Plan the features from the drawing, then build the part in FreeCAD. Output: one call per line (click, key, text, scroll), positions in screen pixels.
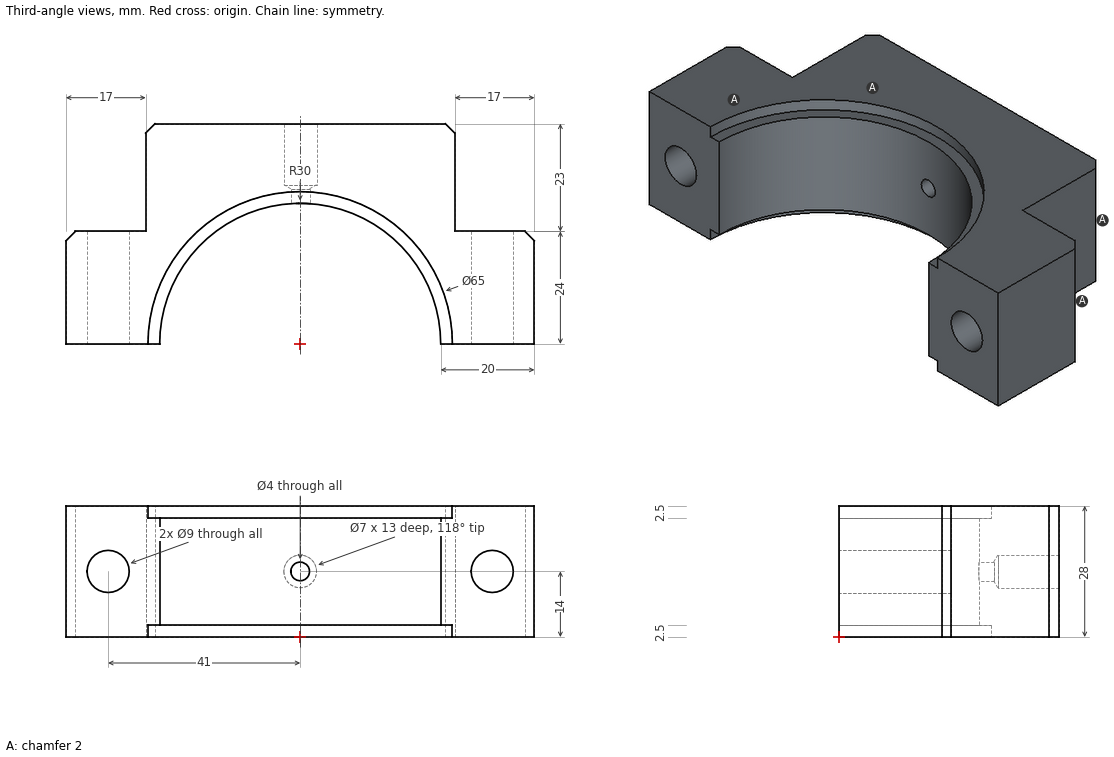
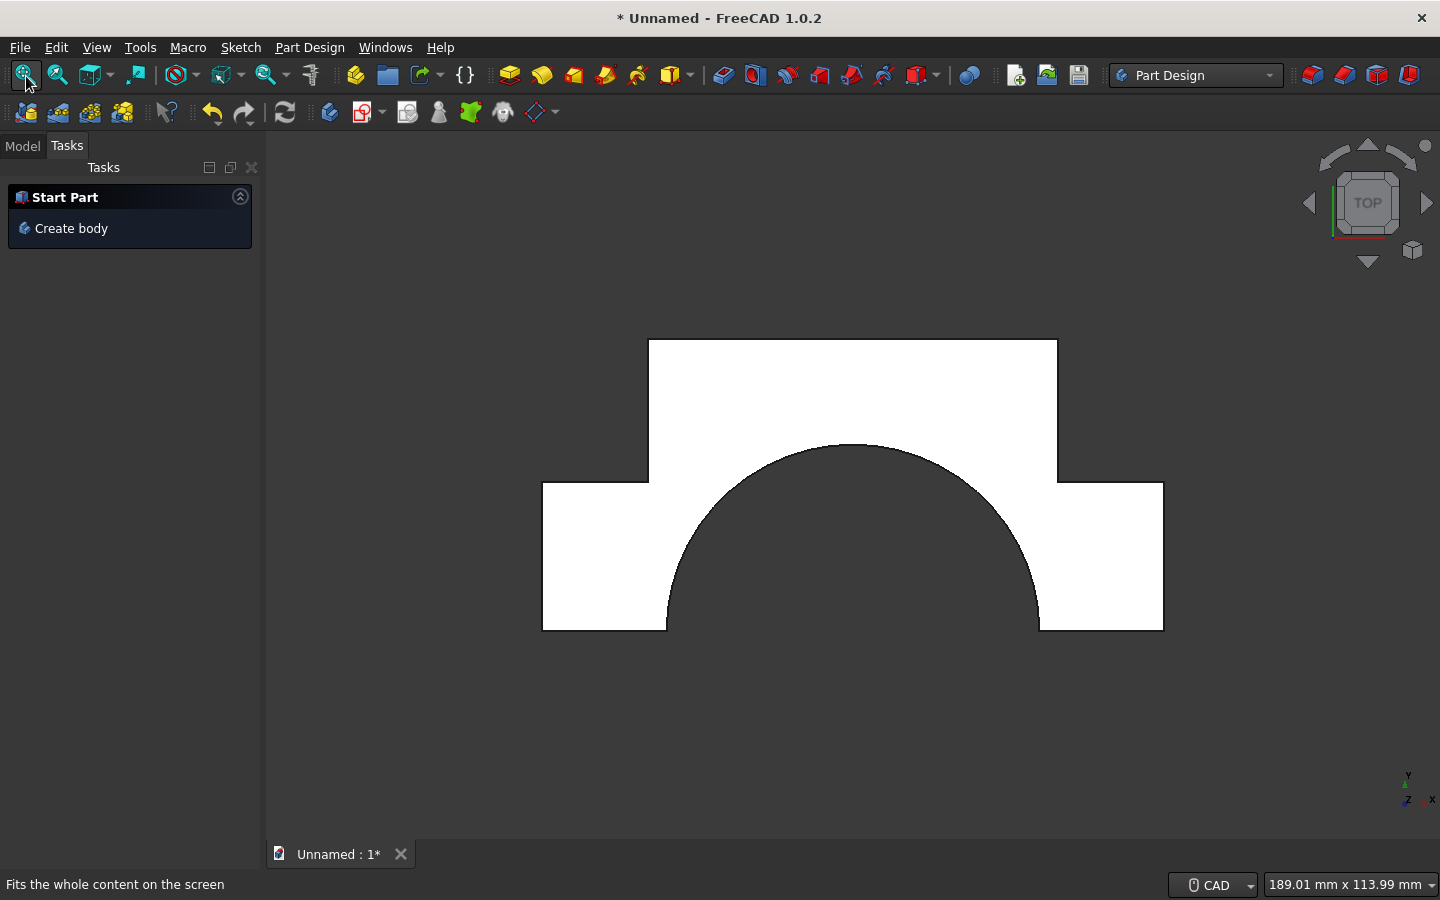
key(1)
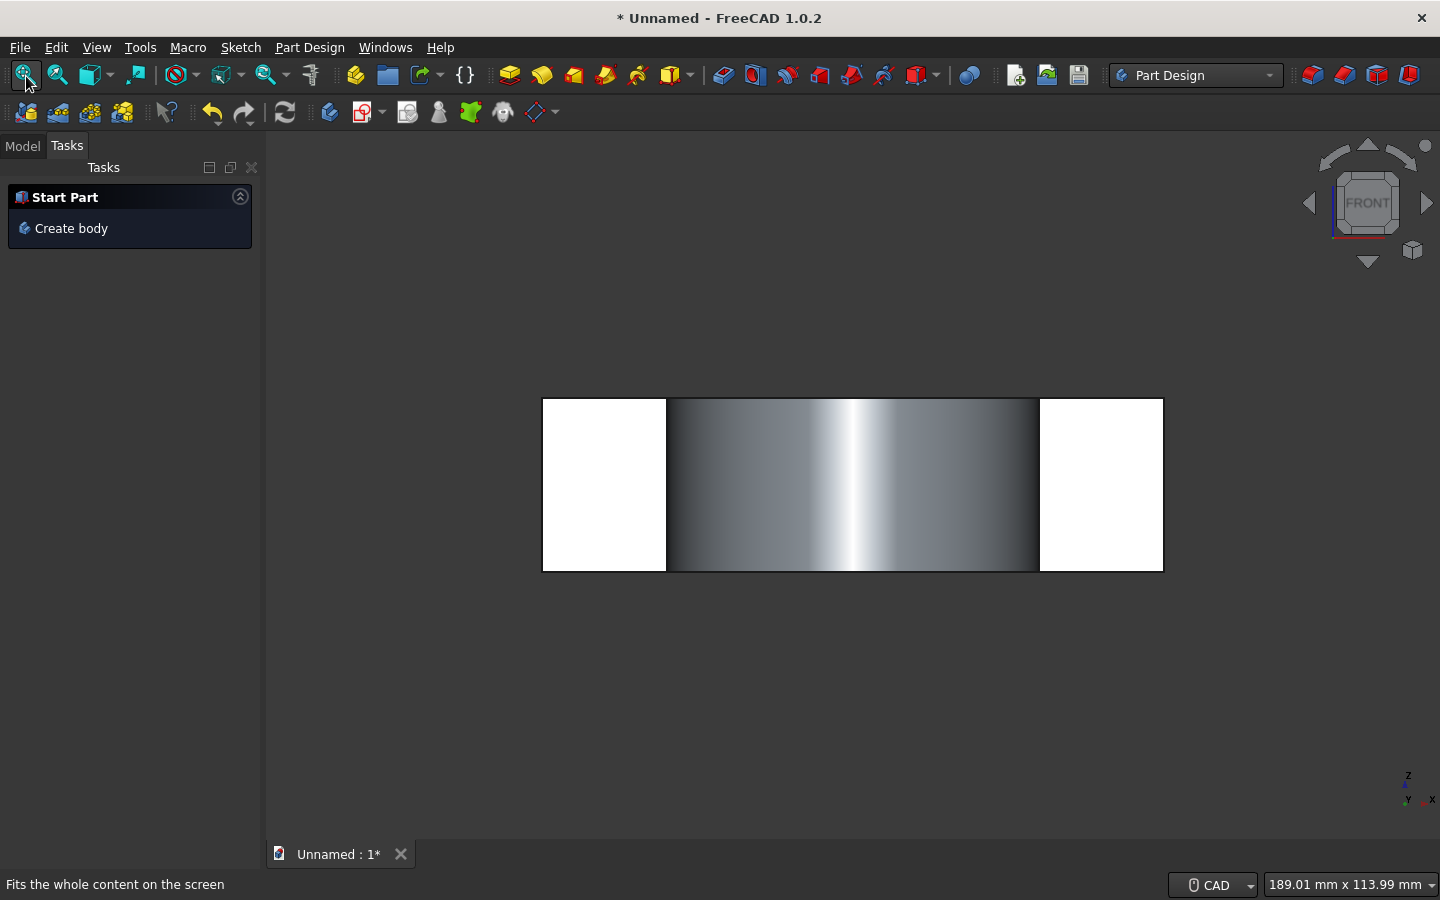
key(3)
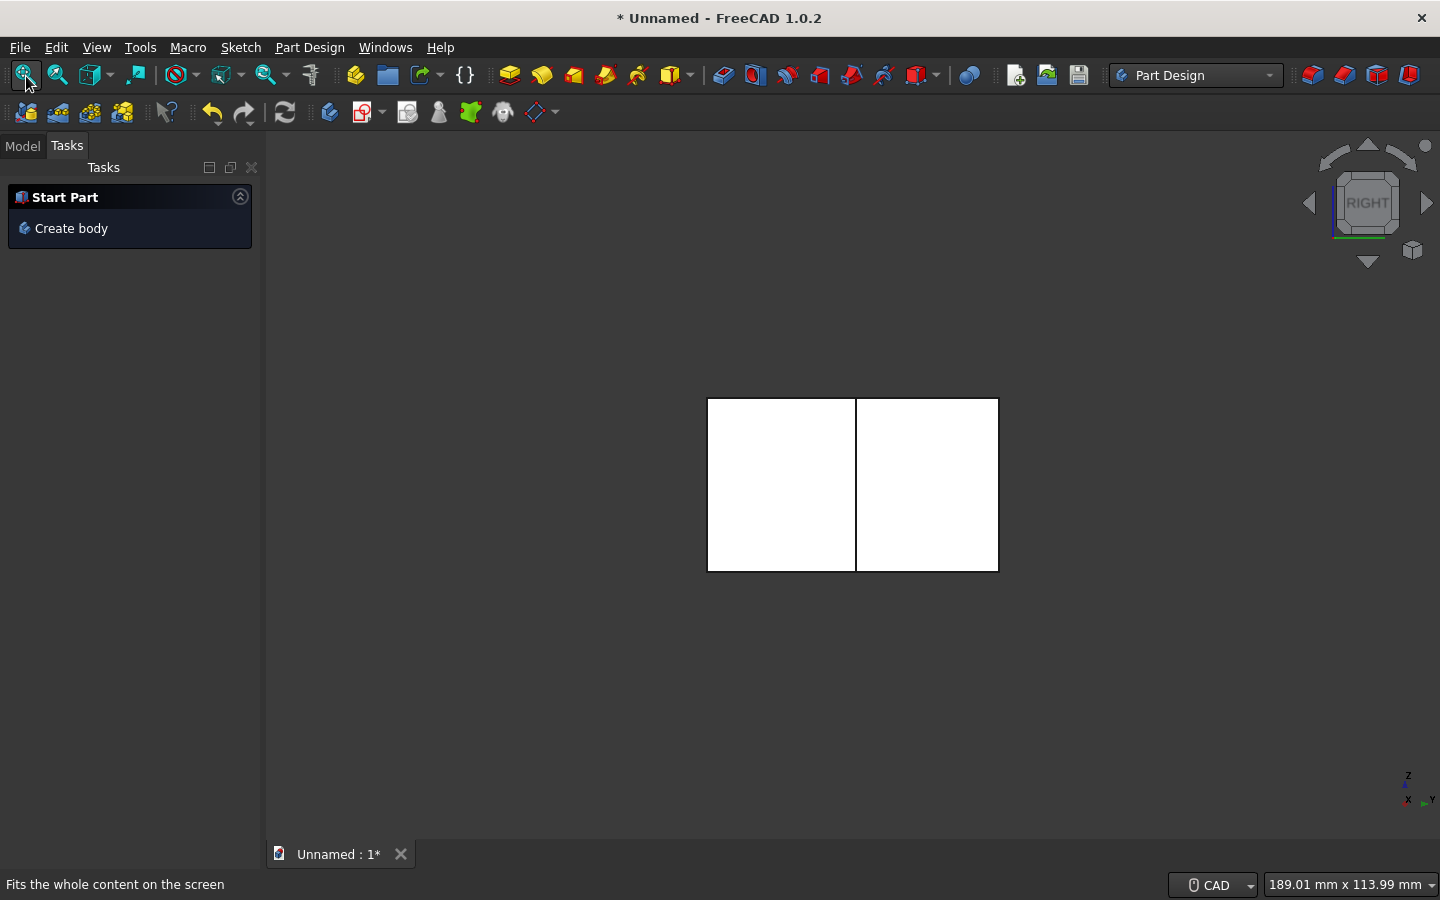
click(26, 76)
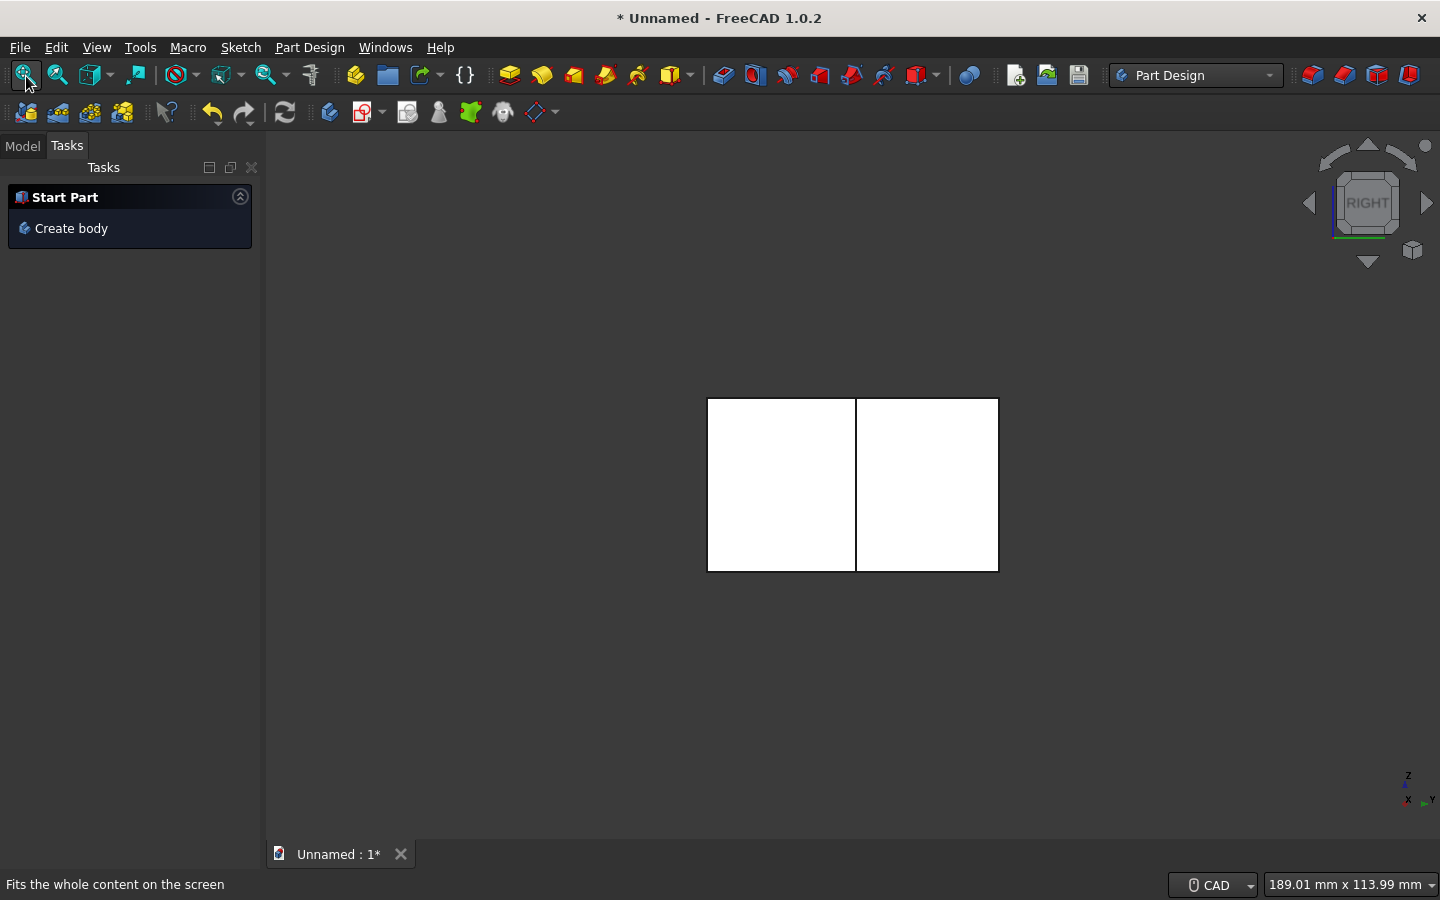
click(999, 484)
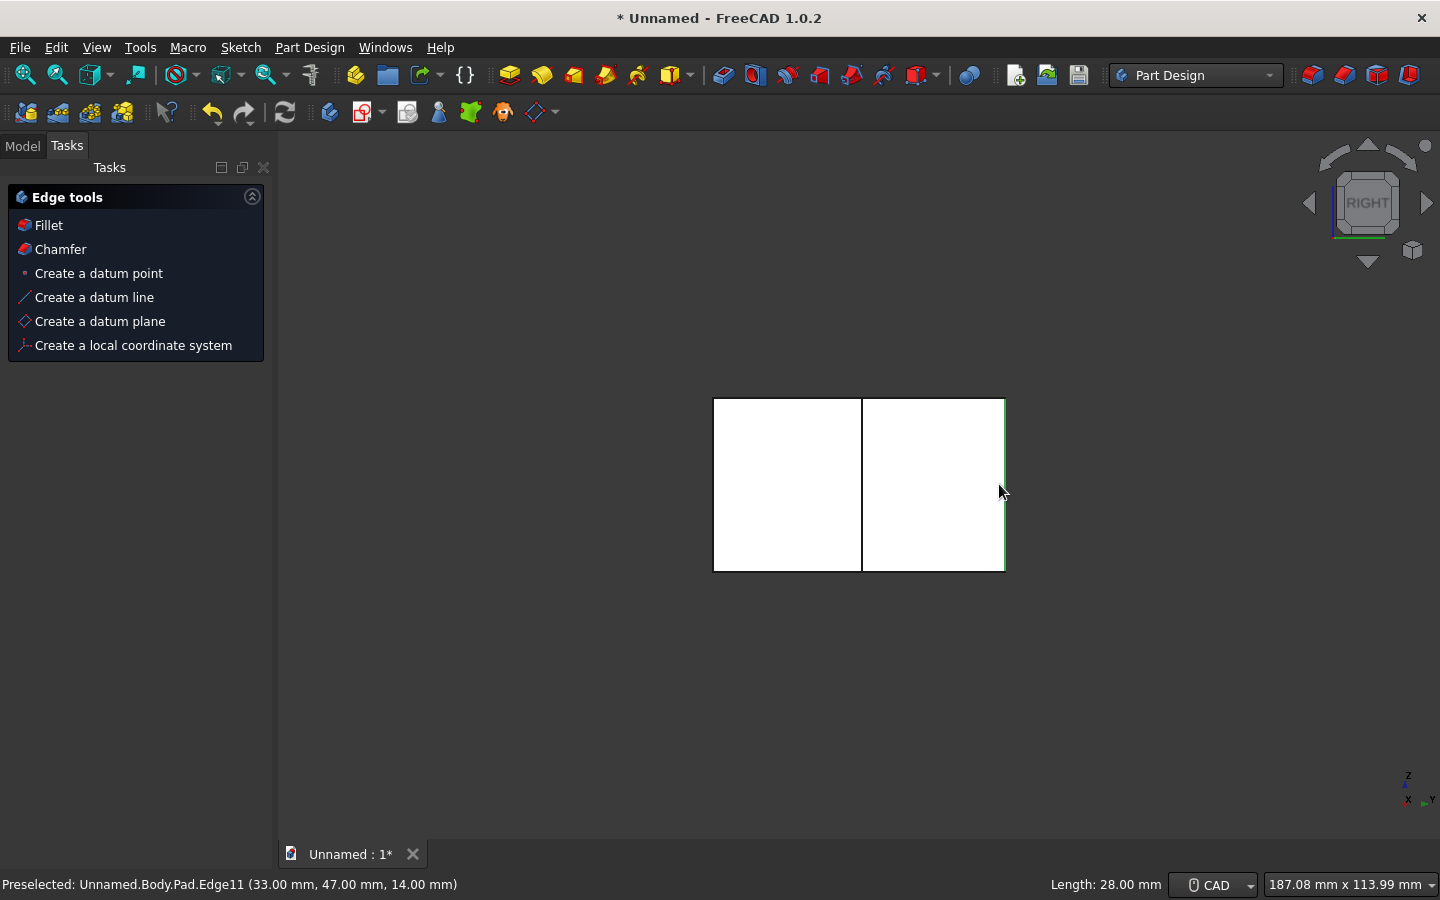
click(862, 484, ctrl)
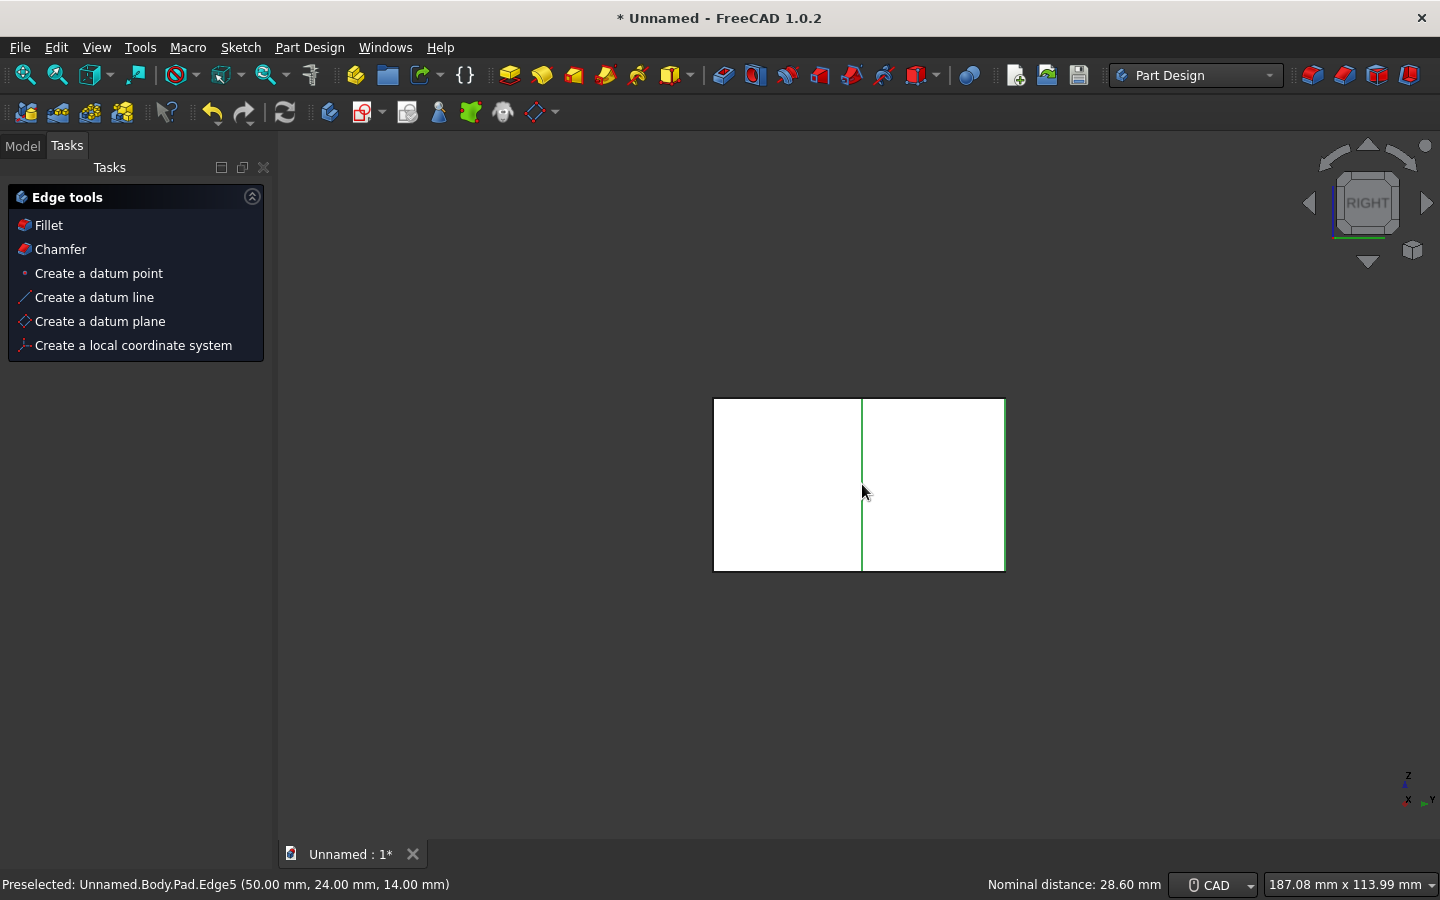
key(5)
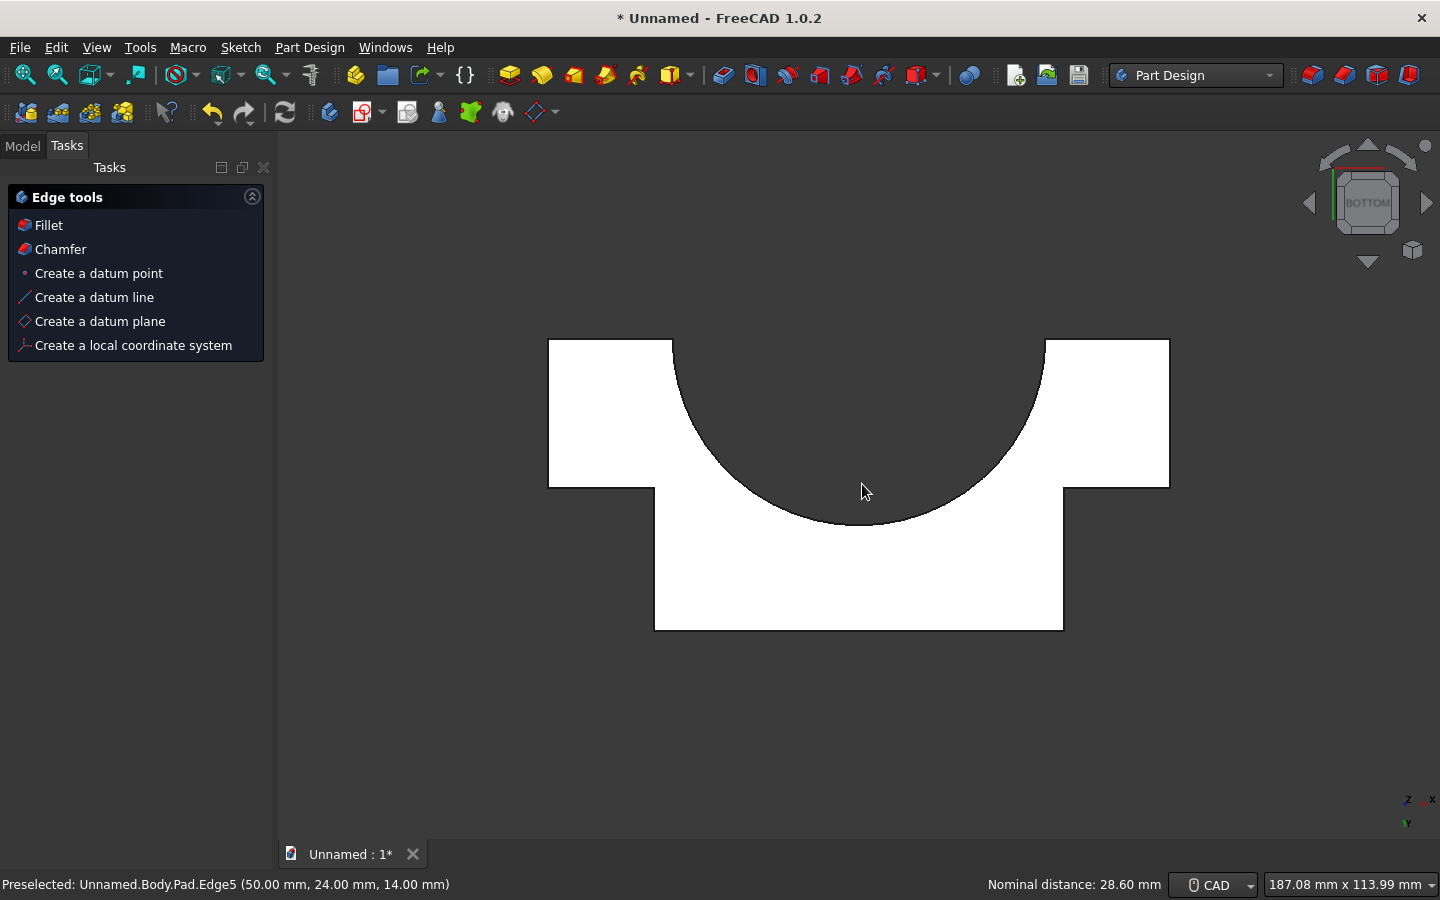
key(4)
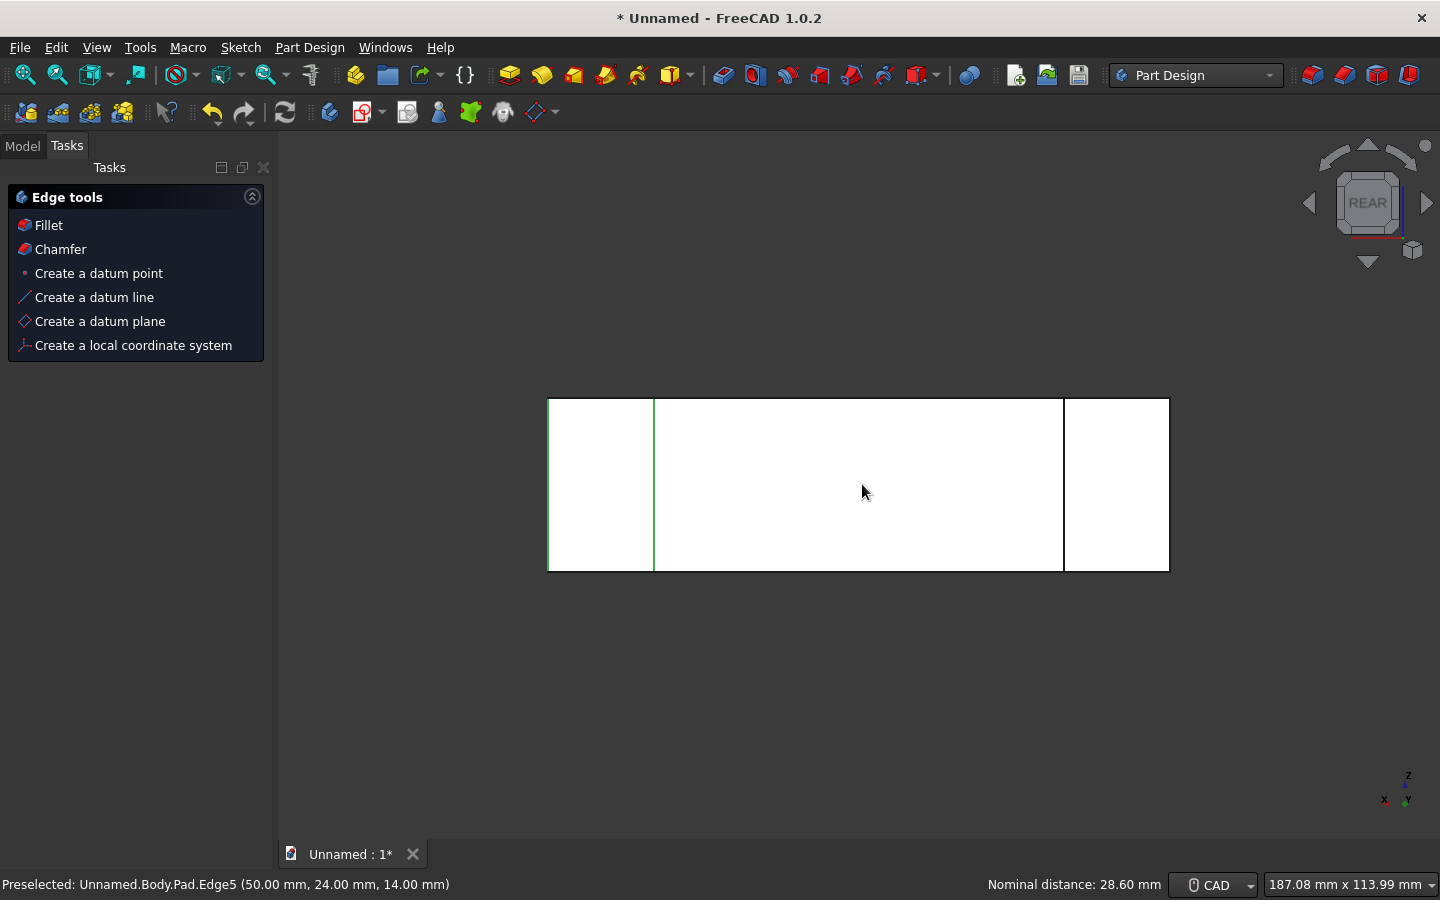
click(1170, 484, ctrl)